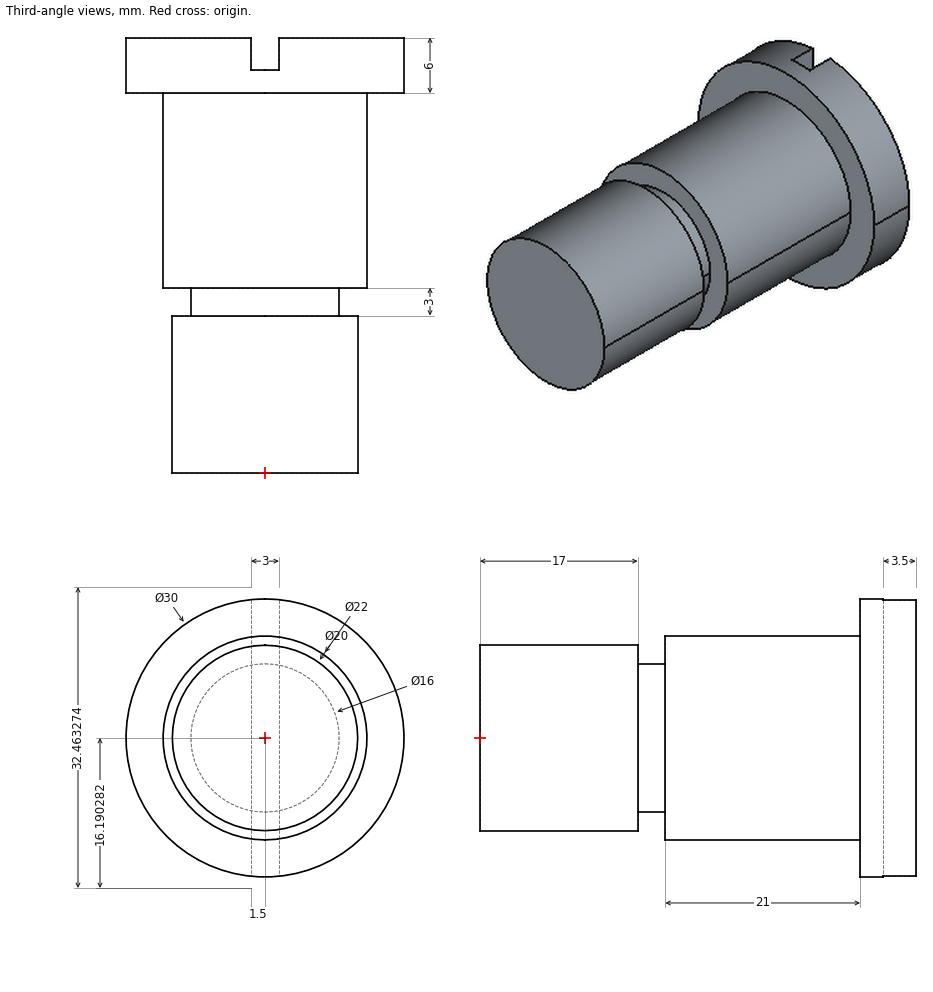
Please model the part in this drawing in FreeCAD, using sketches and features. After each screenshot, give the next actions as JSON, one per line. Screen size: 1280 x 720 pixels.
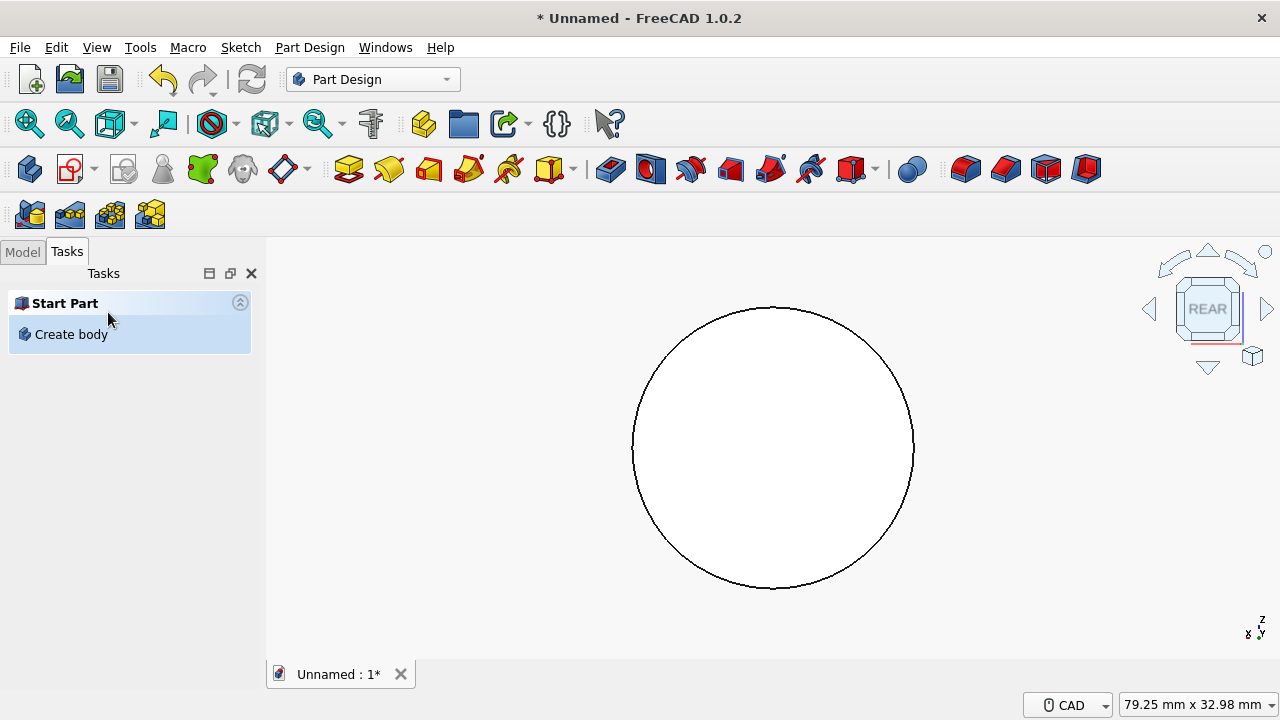
{"action": "left_click", "coordinate": [773, 447]}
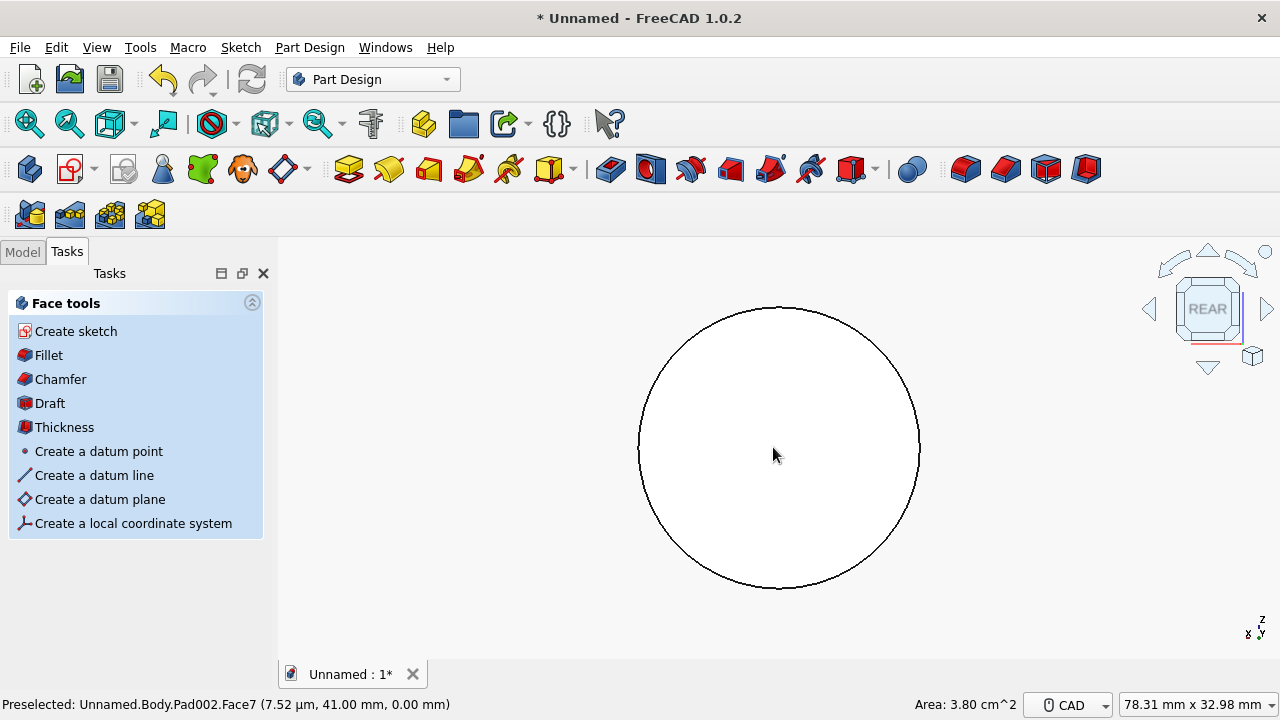
{"action": "left_click", "coordinate": [70, 170]}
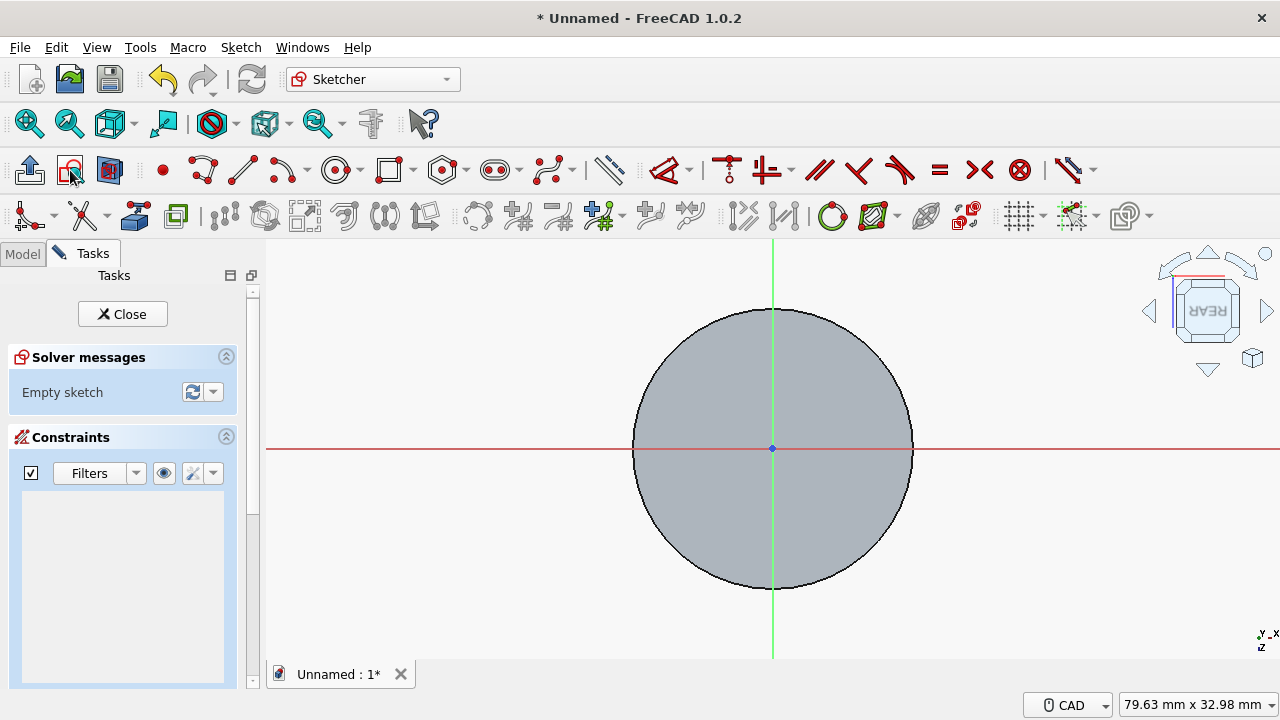
{"action": "scroll", "coordinate": [565, 449], "scroll_direction": "down", "scroll_amount": 2}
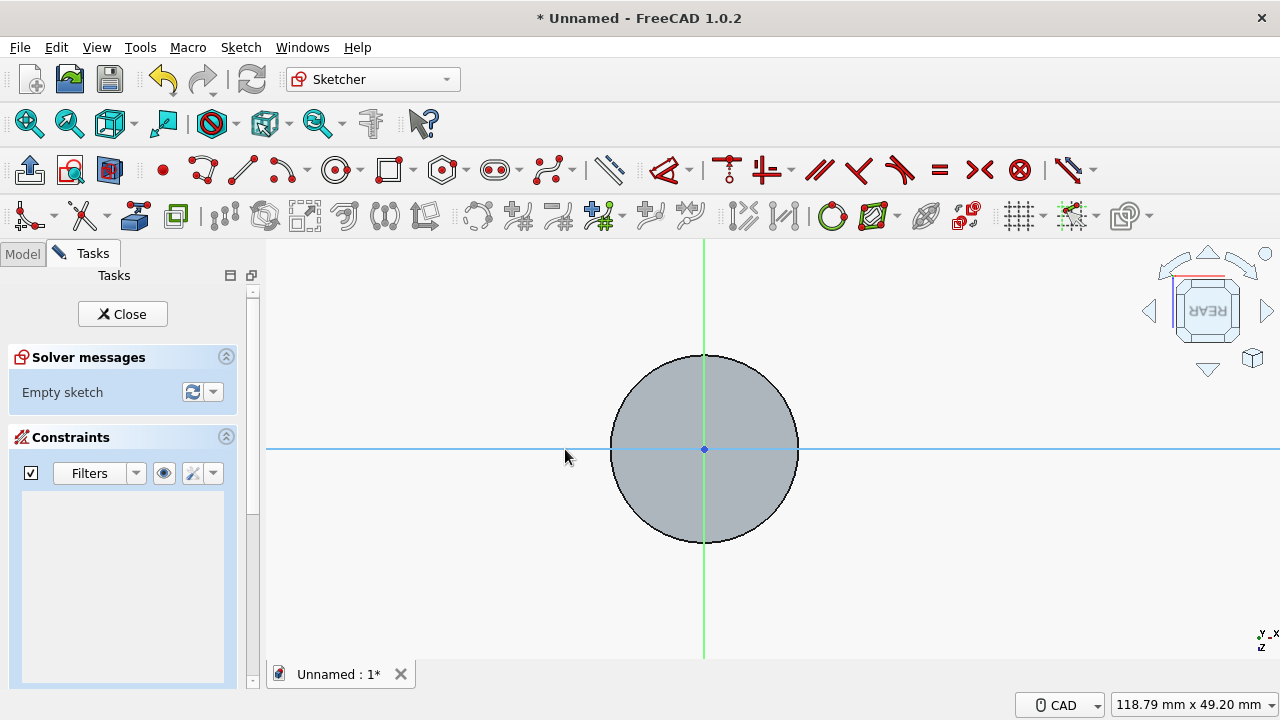
{"action": "left_click", "coordinate": [336, 170]}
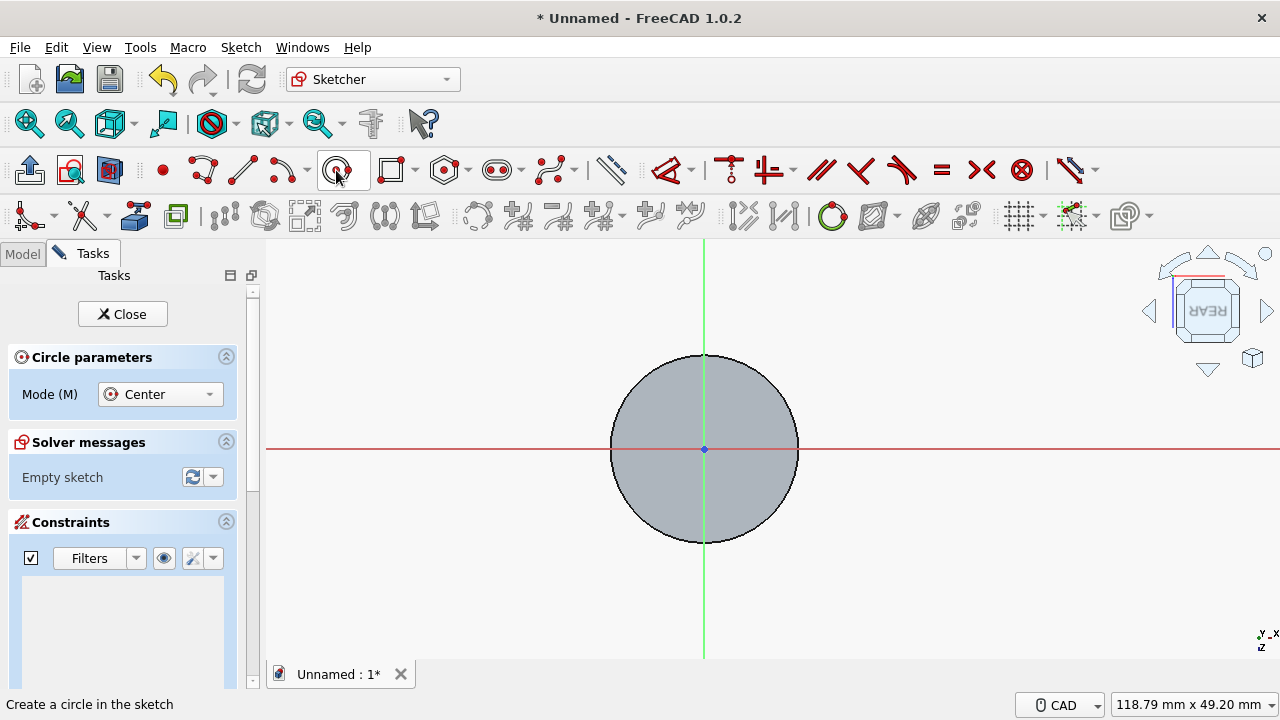
{"action": "left_click", "coordinate": [704, 449]}
{"action": "mouse_move", "coordinate": [795, 359]}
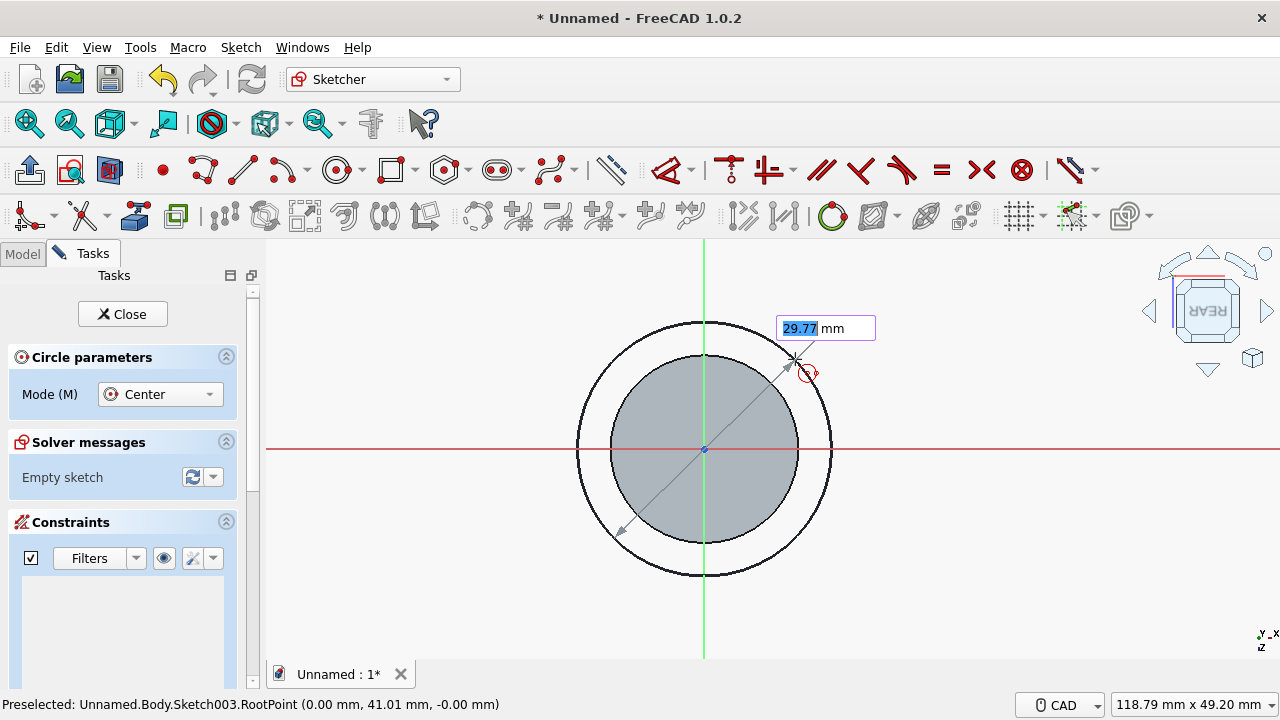
{"action": "type", "text": "30"}
{"action": "key", "text": "Return"}
{"action": "key", "text": "Escape"}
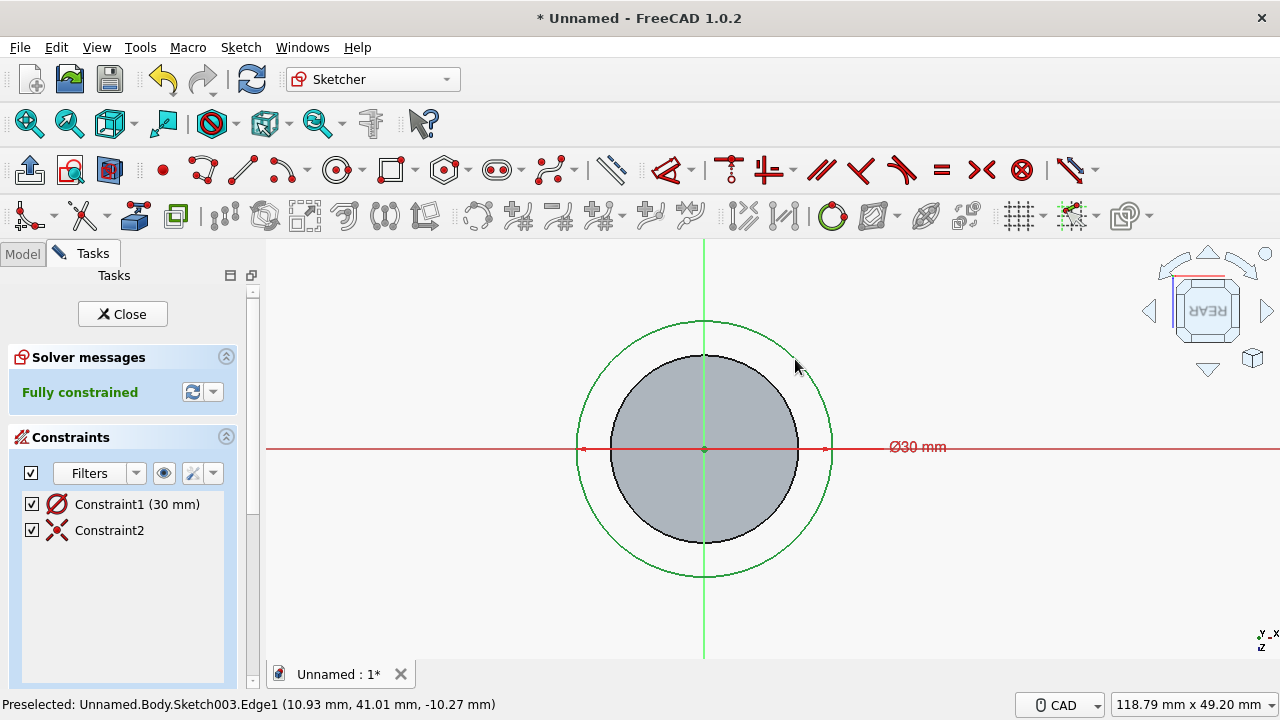
{"action": "left_click", "coordinate": [123, 314]}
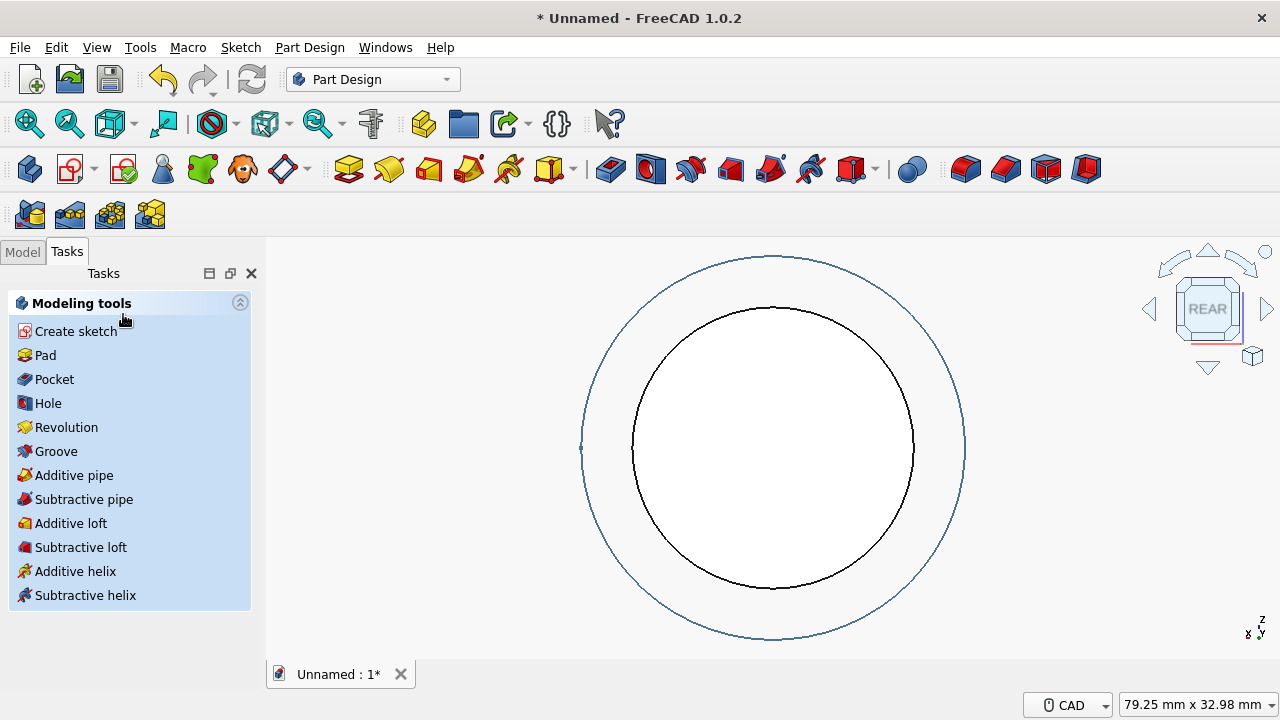
{"action": "left_click", "coordinate": [350, 170]}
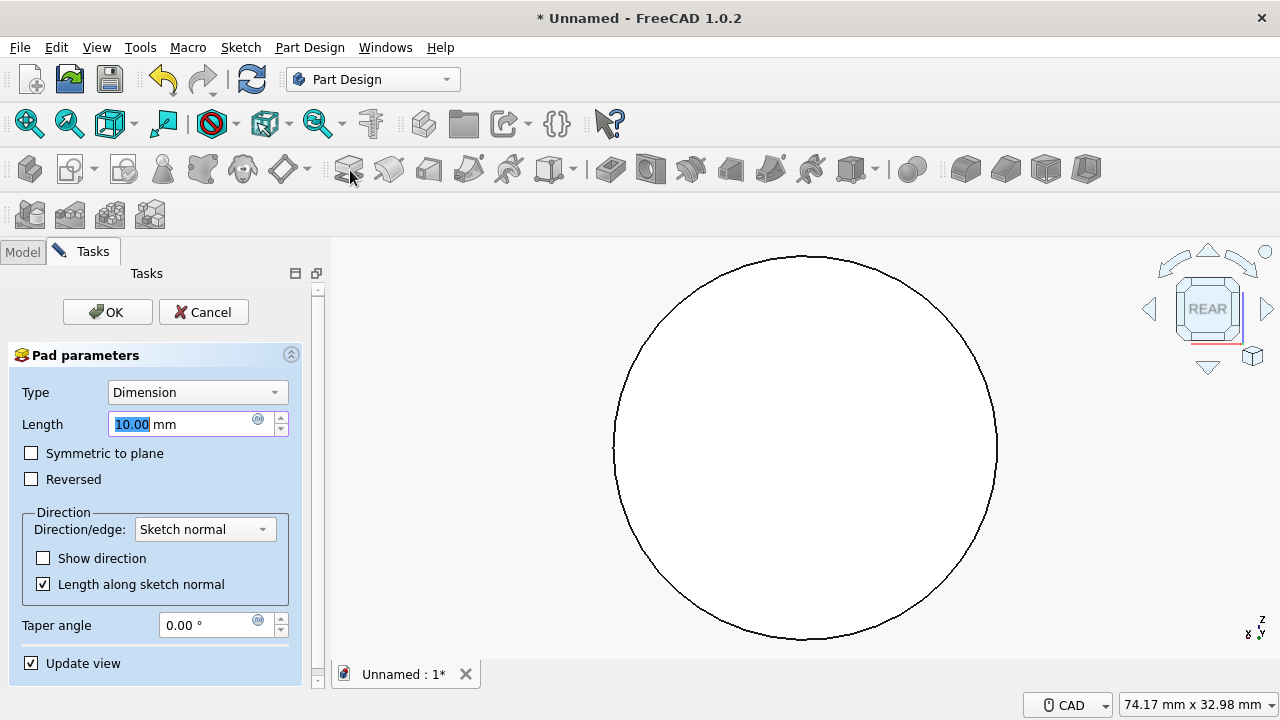
{"action": "type", "text": "6"}
{"action": "key", "text": "Tab"}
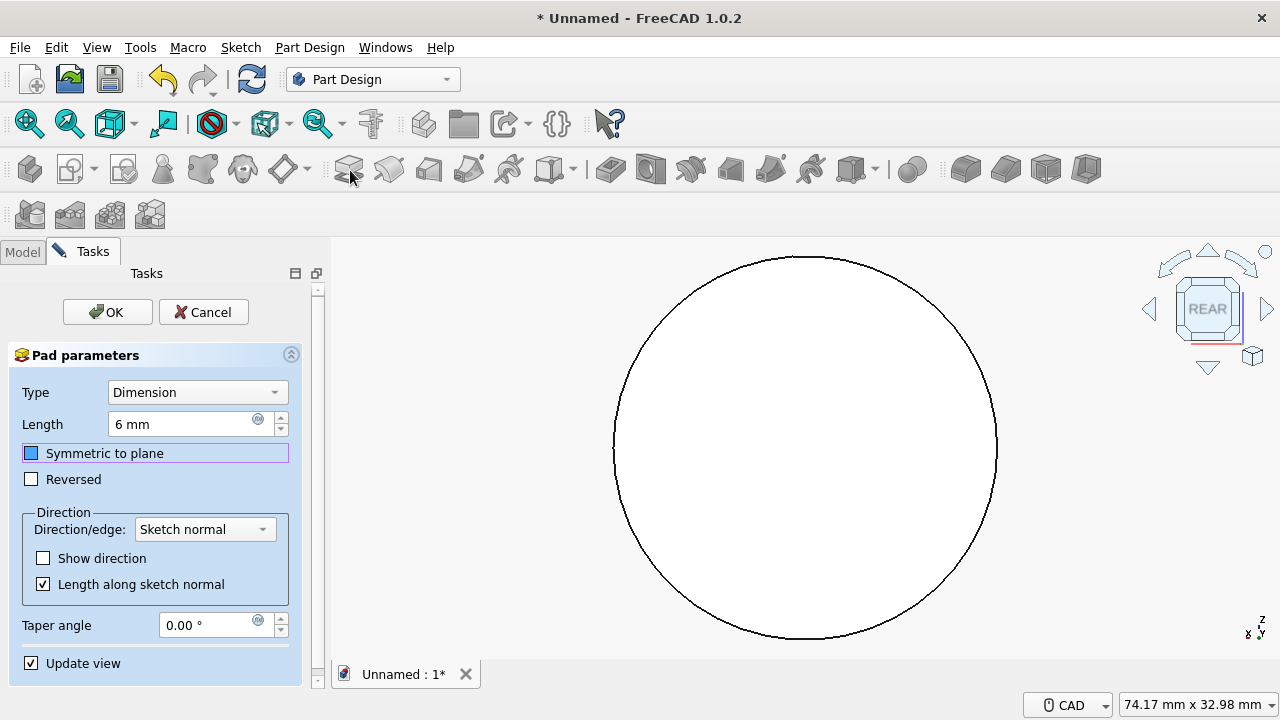
{"action": "left_click", "coordinate": [108, 312]}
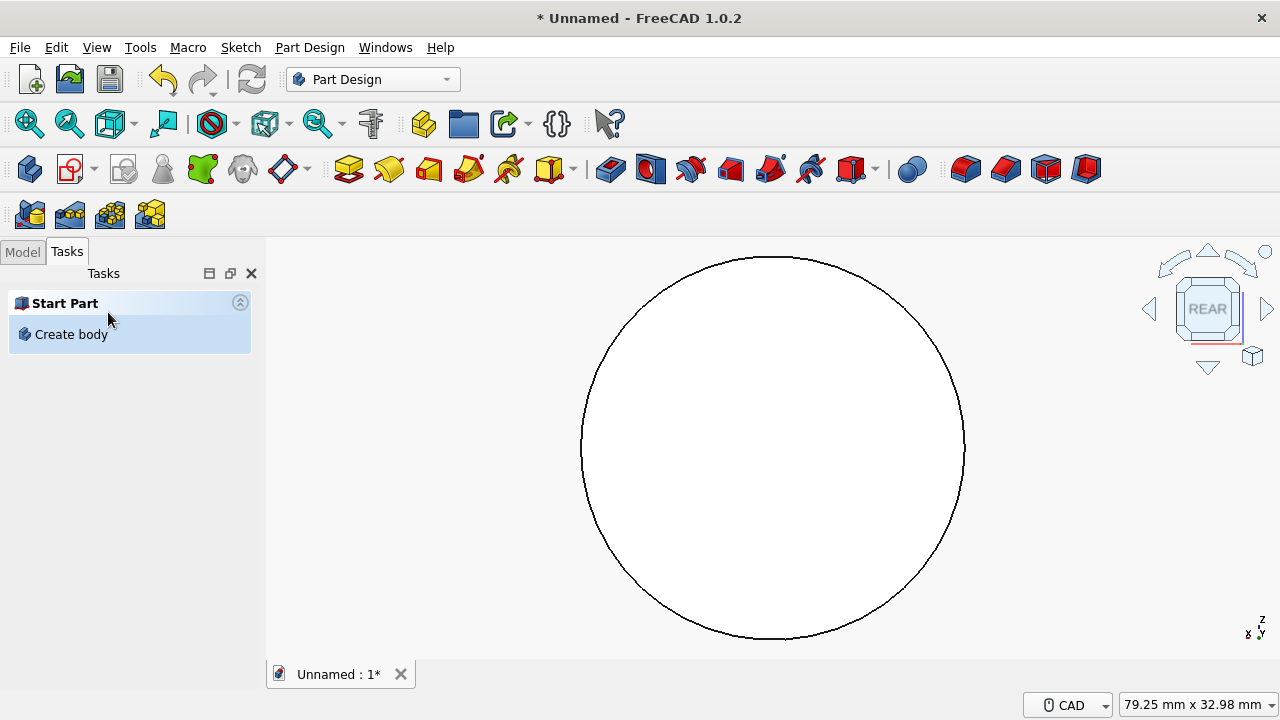
{"action": "left_click", "coordinate": [773, 447]}